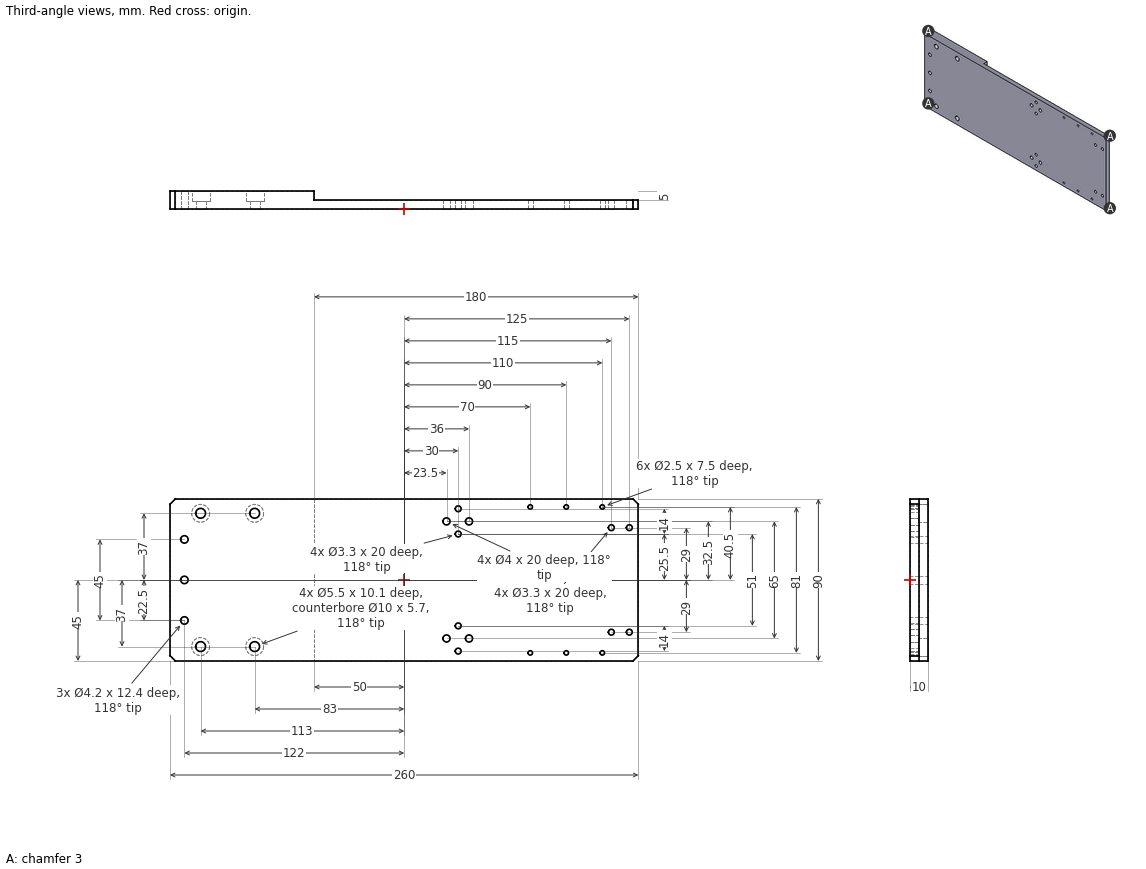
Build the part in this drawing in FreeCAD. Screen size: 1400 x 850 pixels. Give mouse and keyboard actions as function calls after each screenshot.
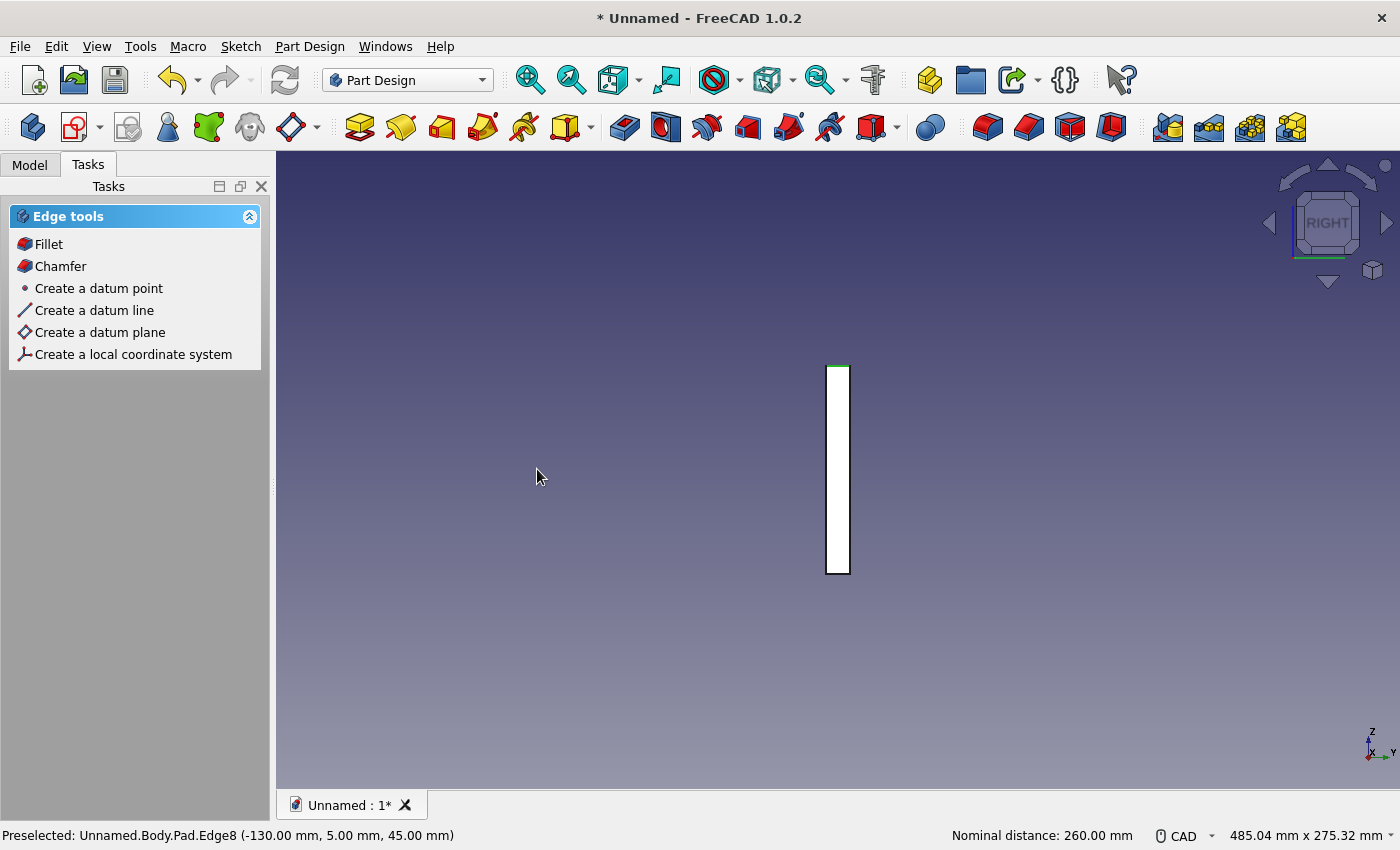
click(531, 80)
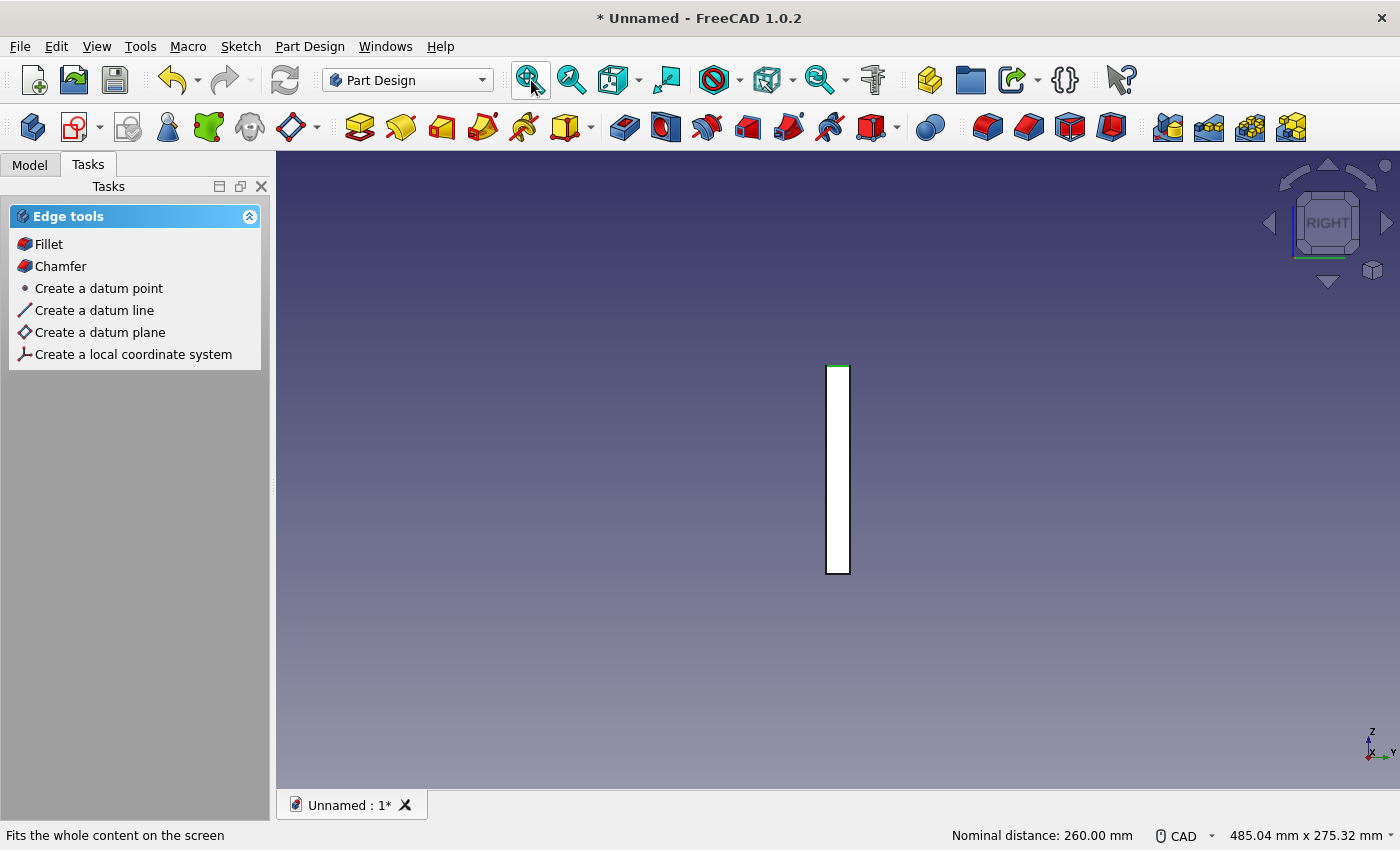
click(838, 573, ctrl)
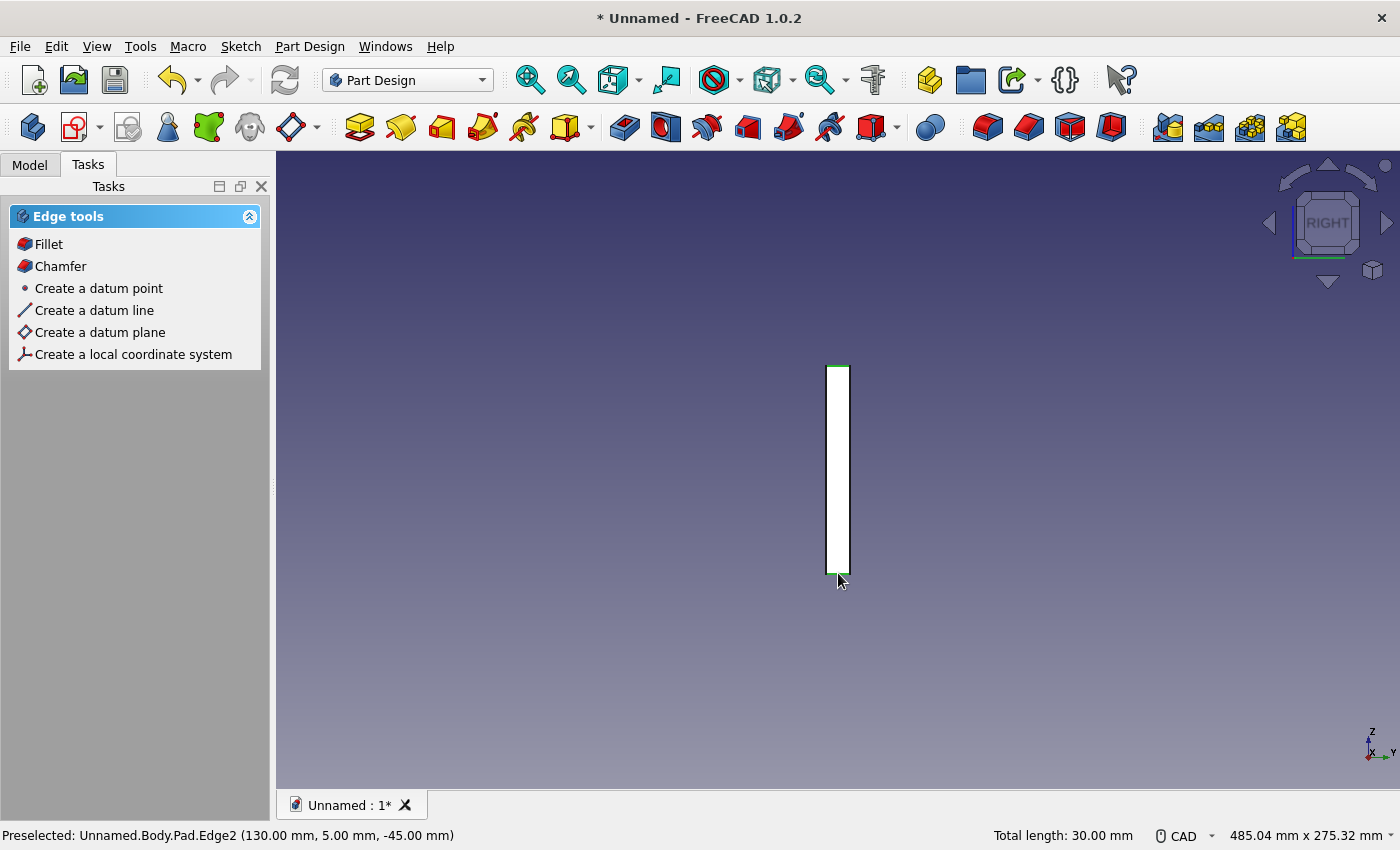
key(5)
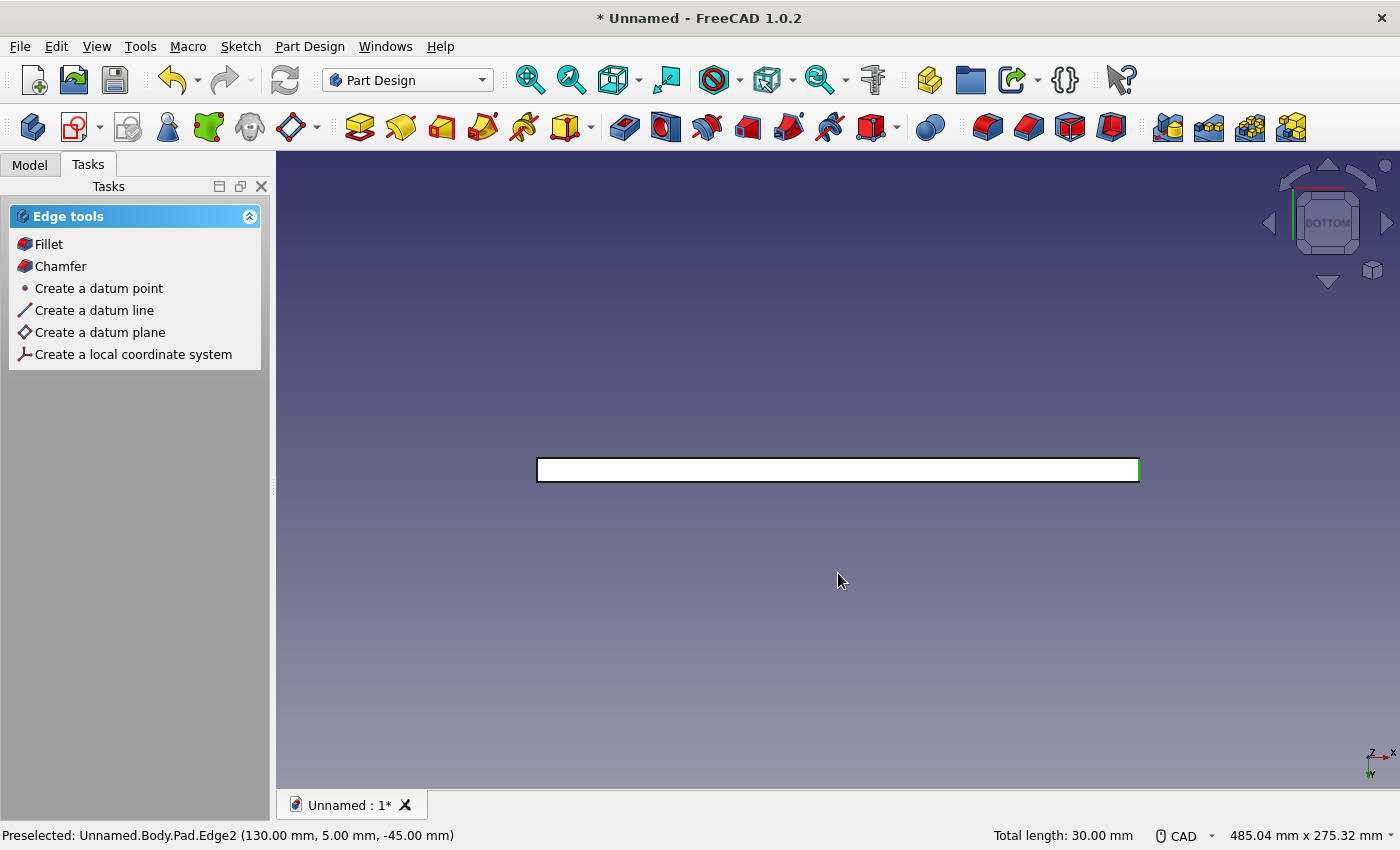
click(537, 469, ctrl)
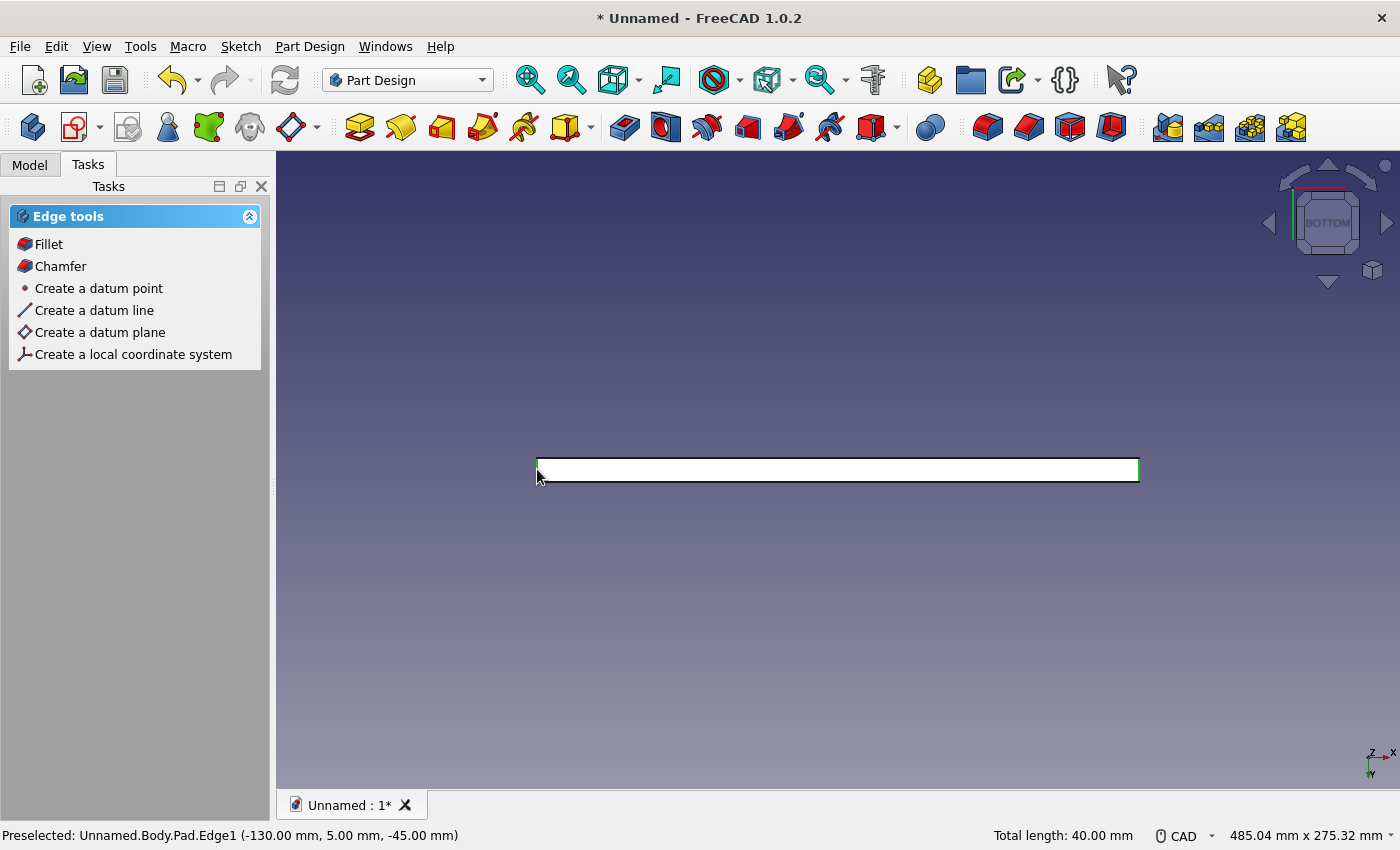
click(1029, 128)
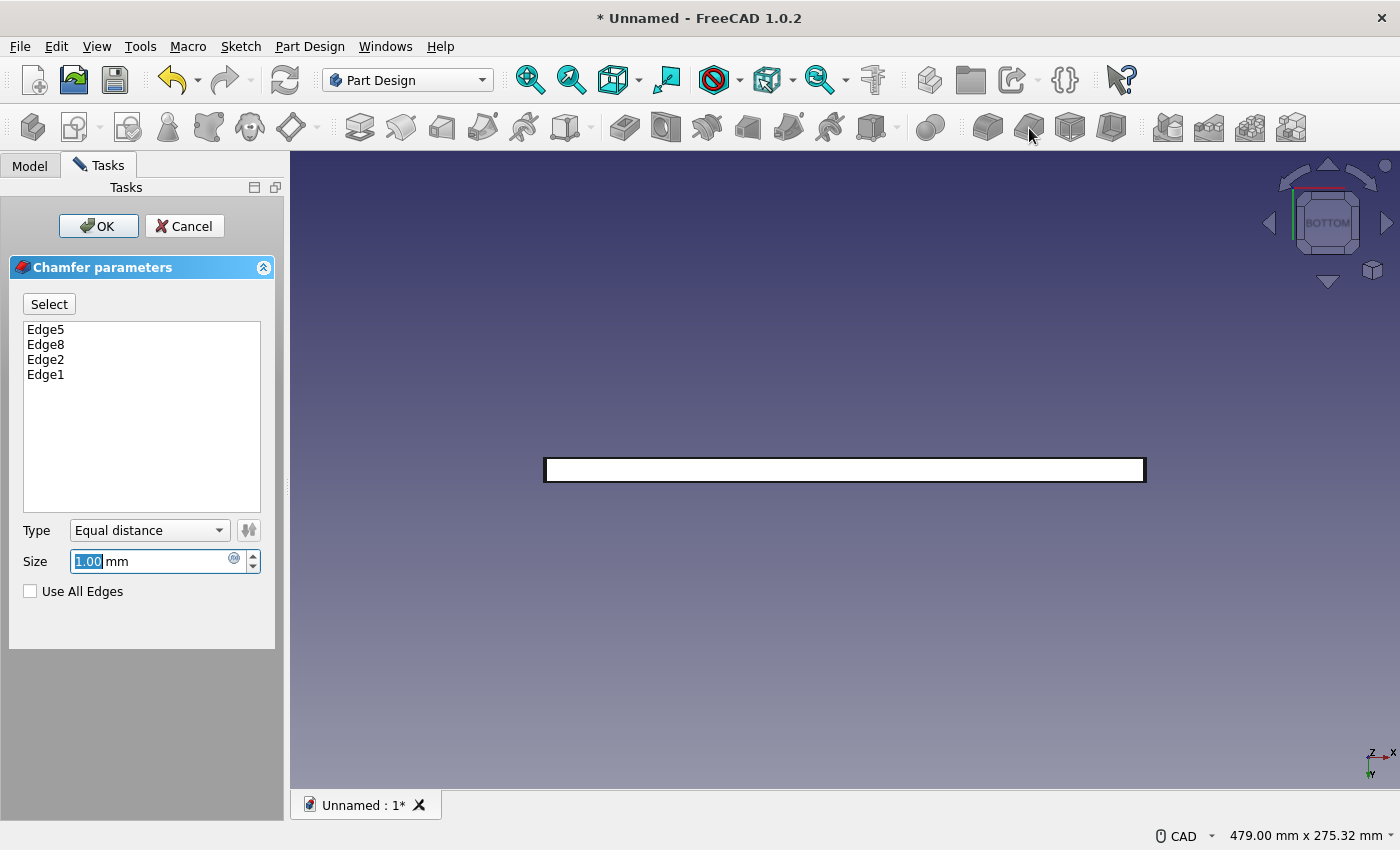
text(3)
key(Tab)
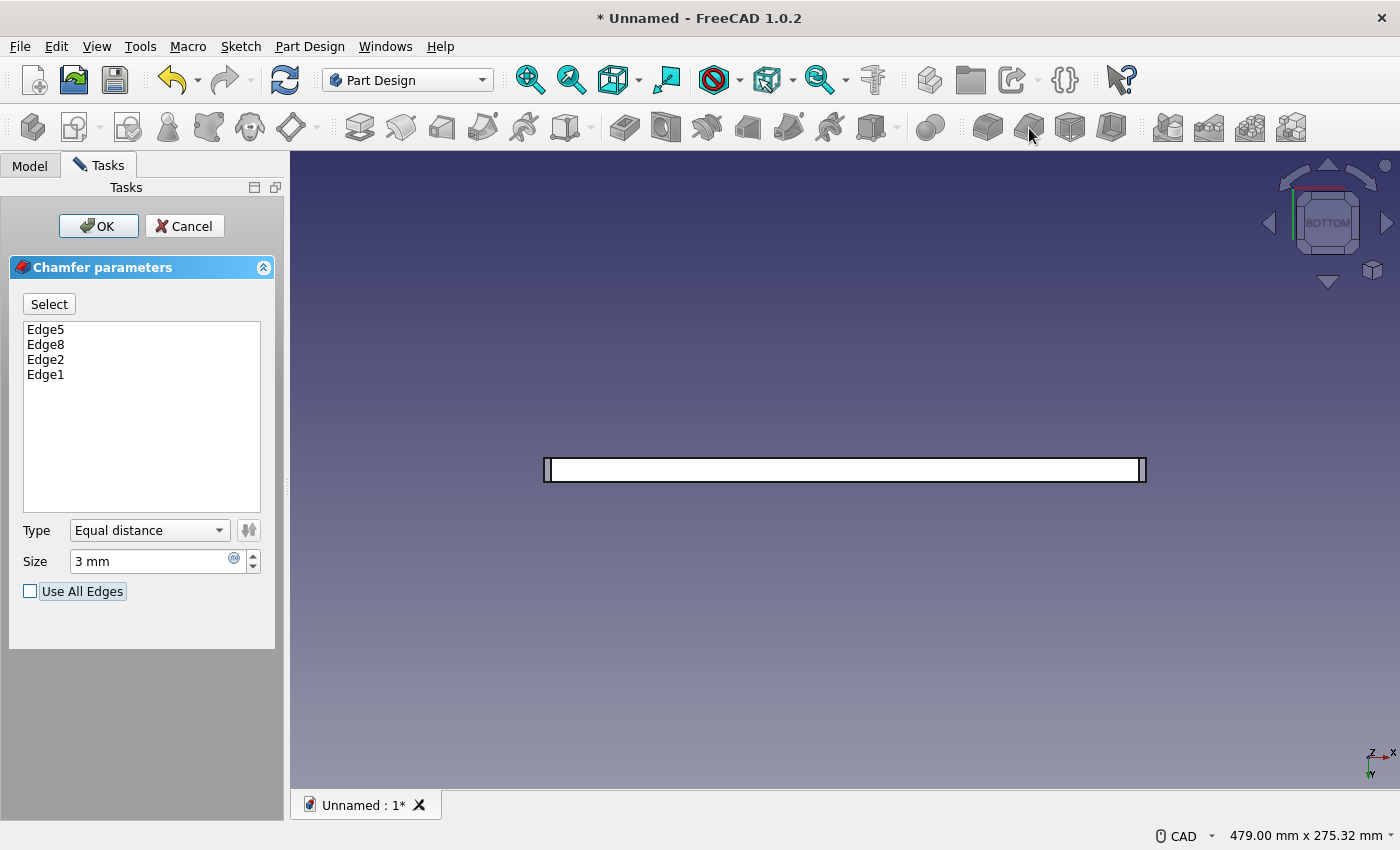
click(99, 226)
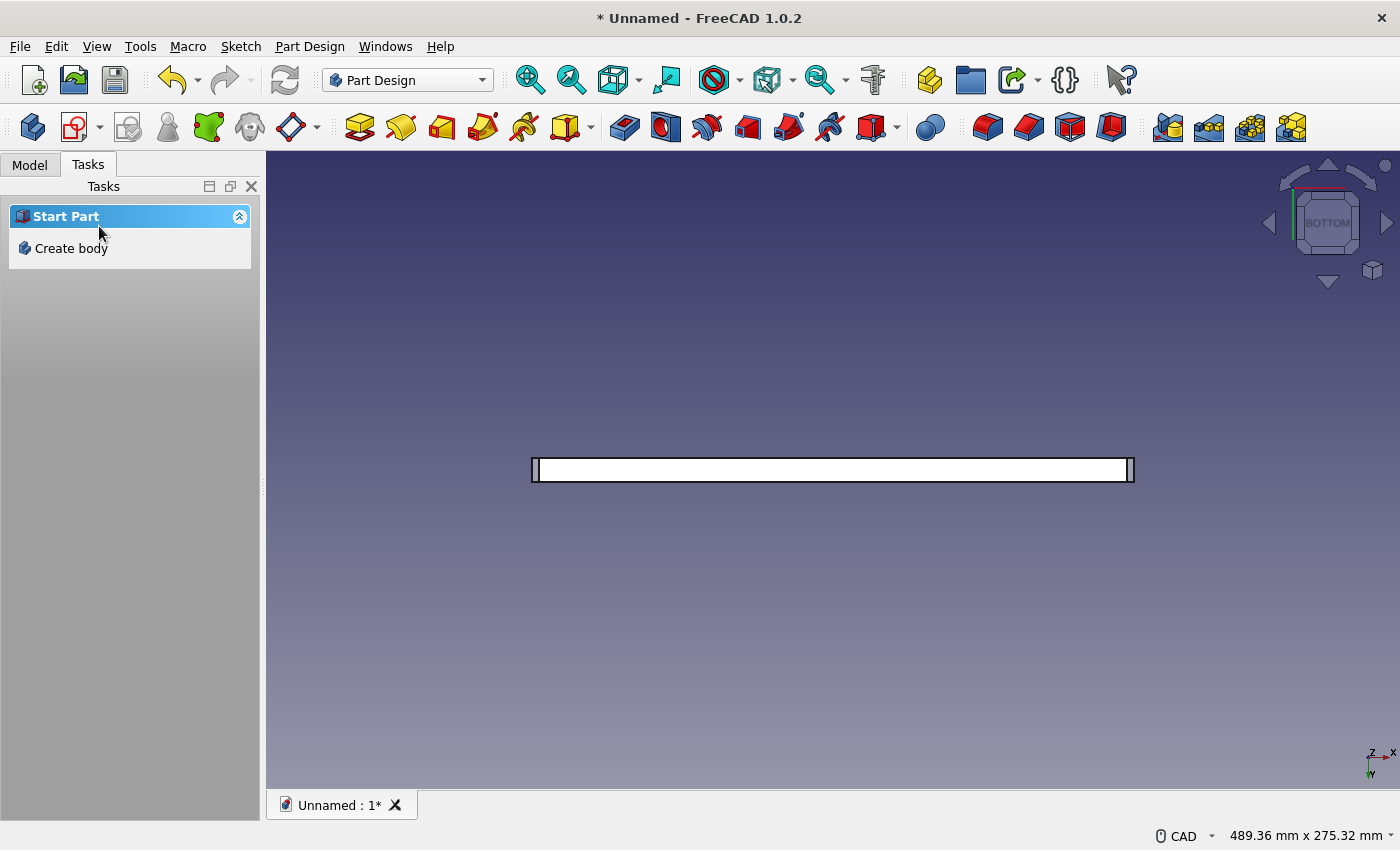
key(4)